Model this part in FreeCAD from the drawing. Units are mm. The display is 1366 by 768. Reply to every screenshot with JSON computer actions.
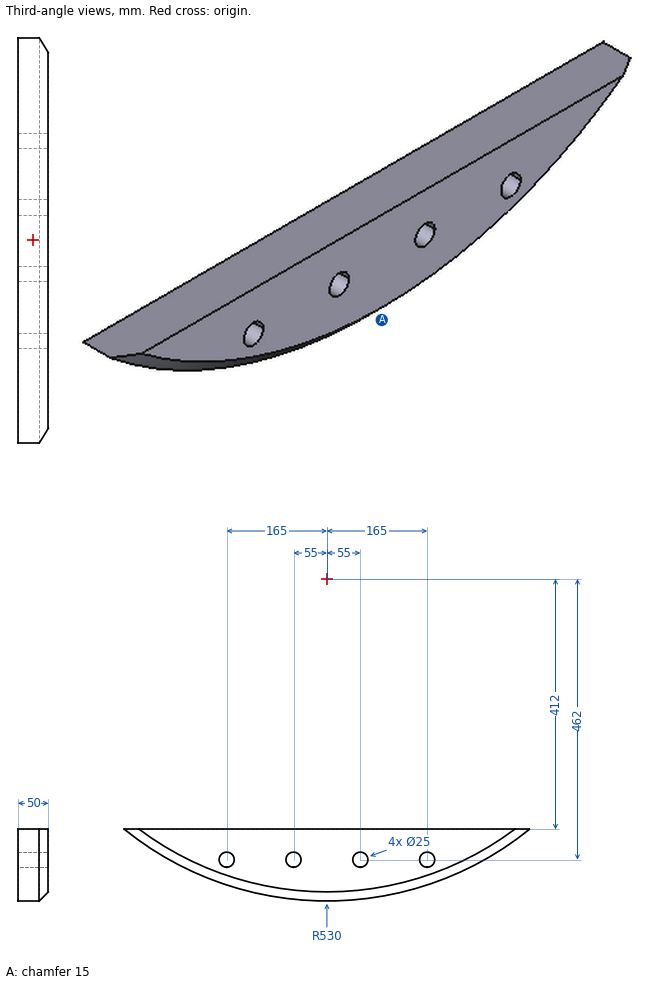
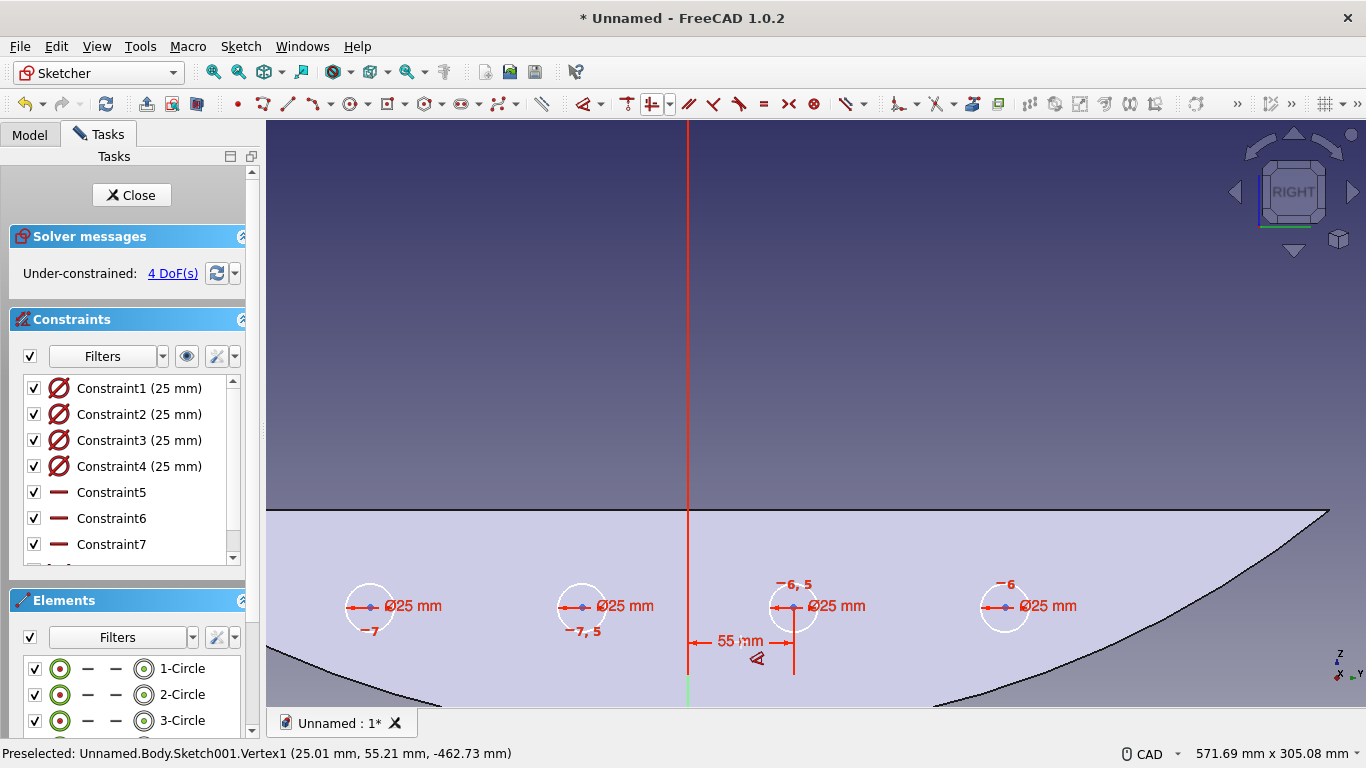
{"action": "left_click", "coordinate": [582, 608]}
{"action": "left_click", "coordinate": [635, 642]}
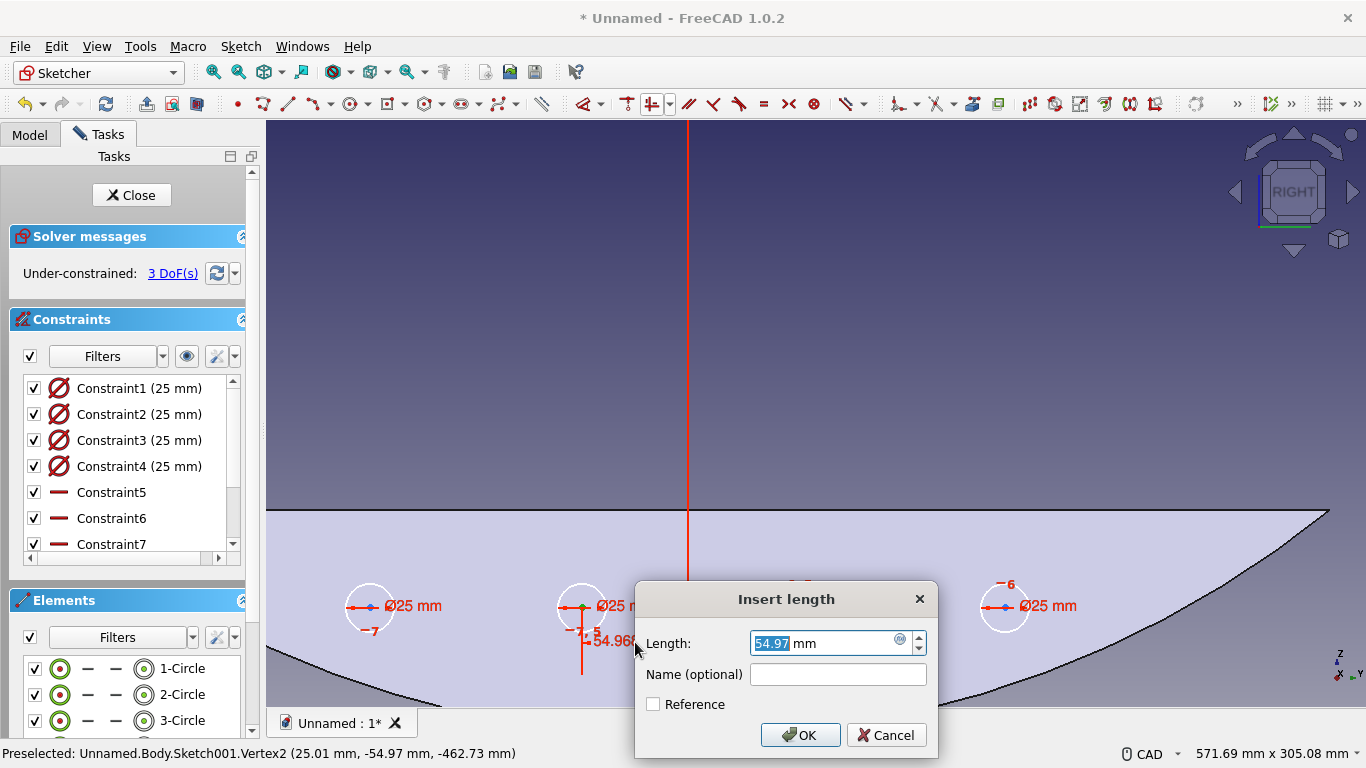
{"action": "type", "text": "55"}
{"action": "key", "text": "Return"}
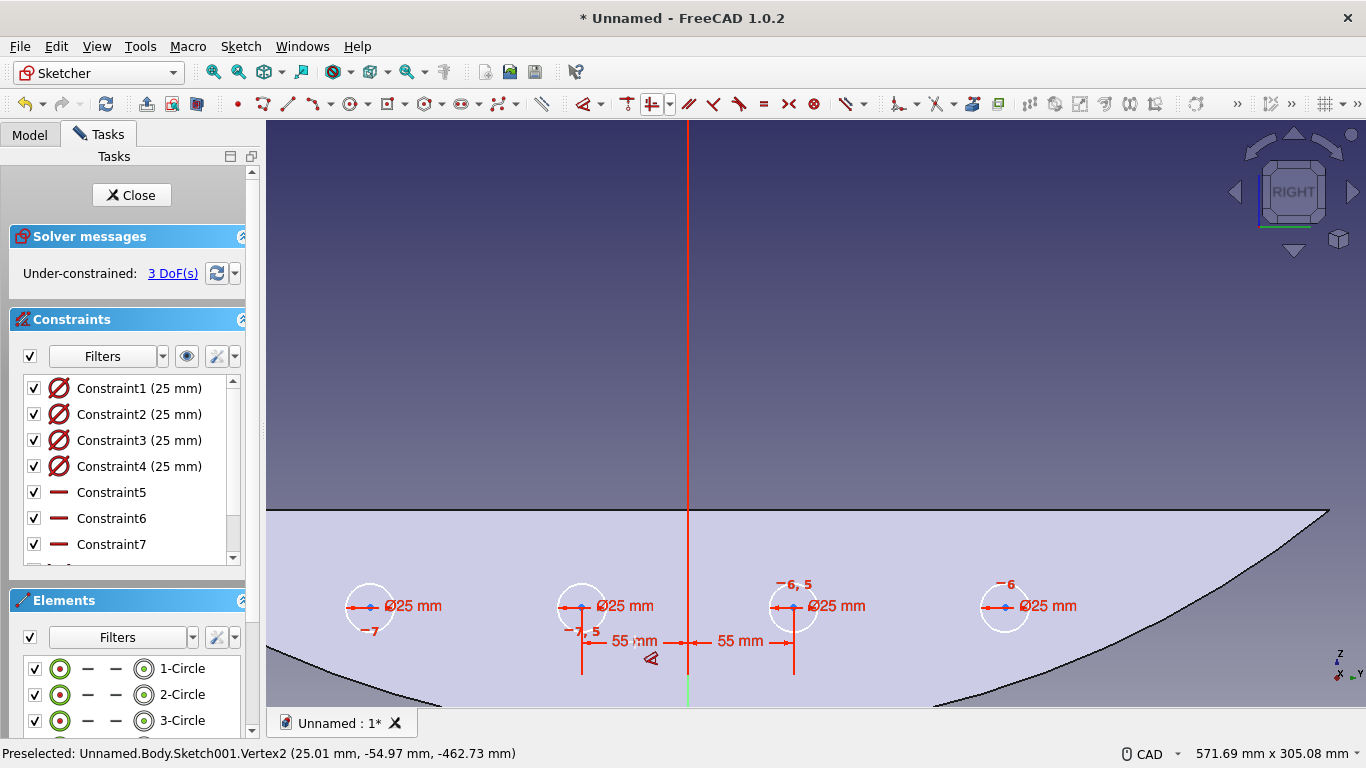
{"action": "left_click", "coordinate": [794, 608]}
{"action": "left_click", "coordinate": [828, 378]}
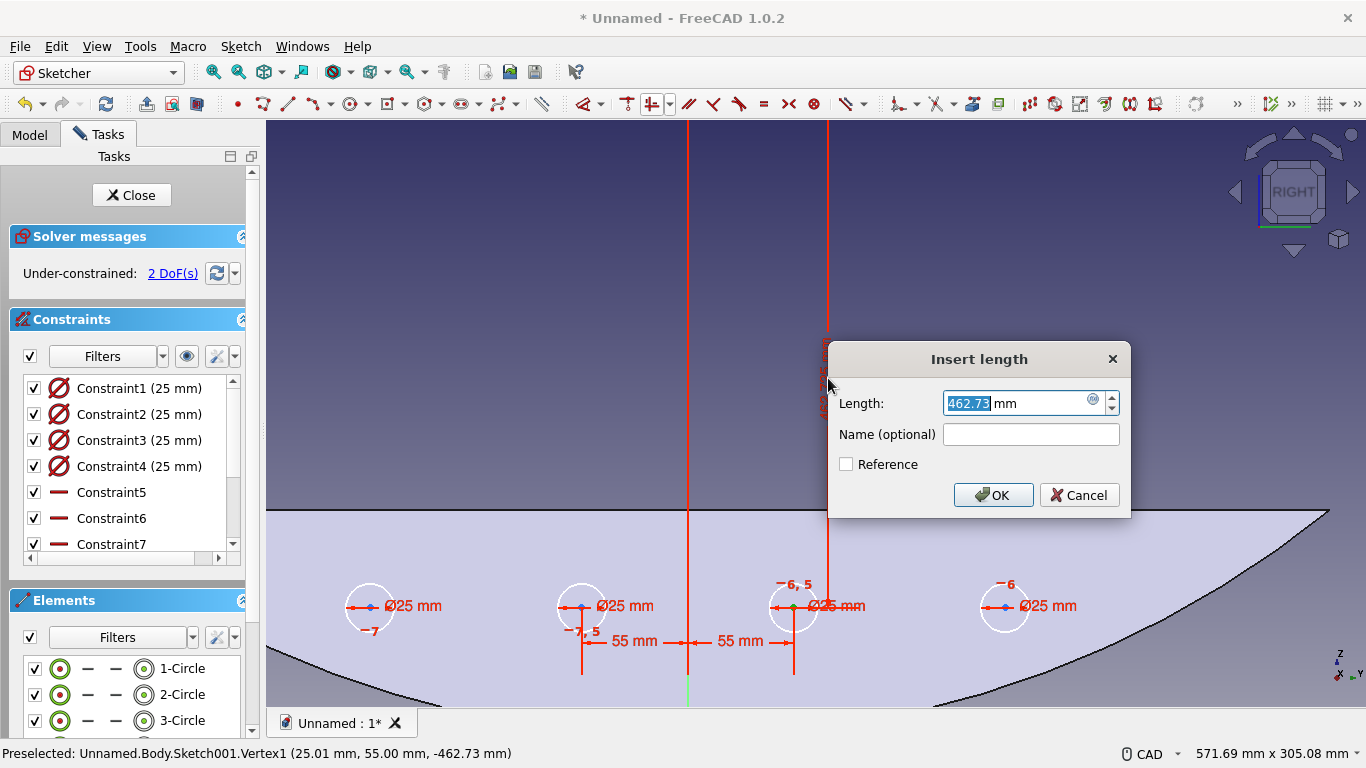
{"action": "type", "text": "462"}
{"action": "key", "text": "Return"}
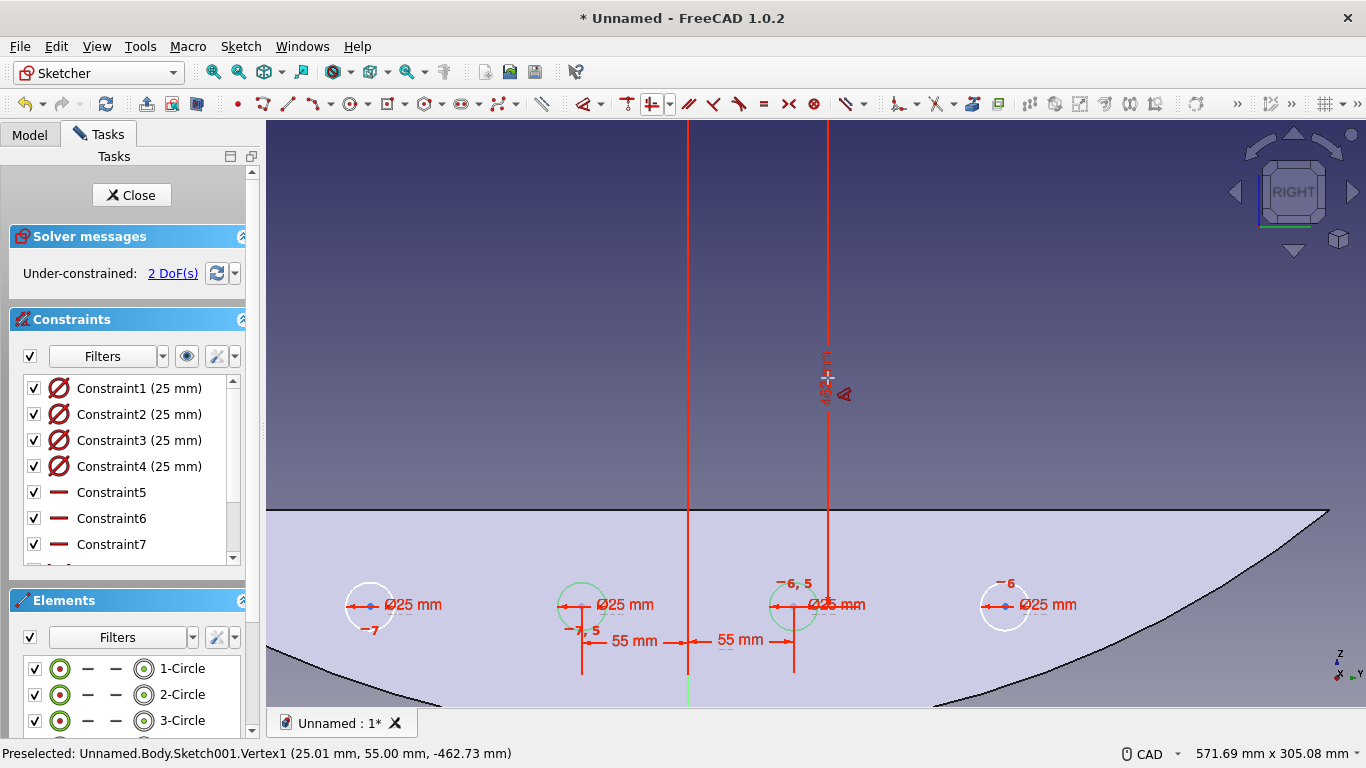
{"action": "left_click", "coordinate": [1005, 607]}
{"action": "left_click", "coordinate": [846, 641]}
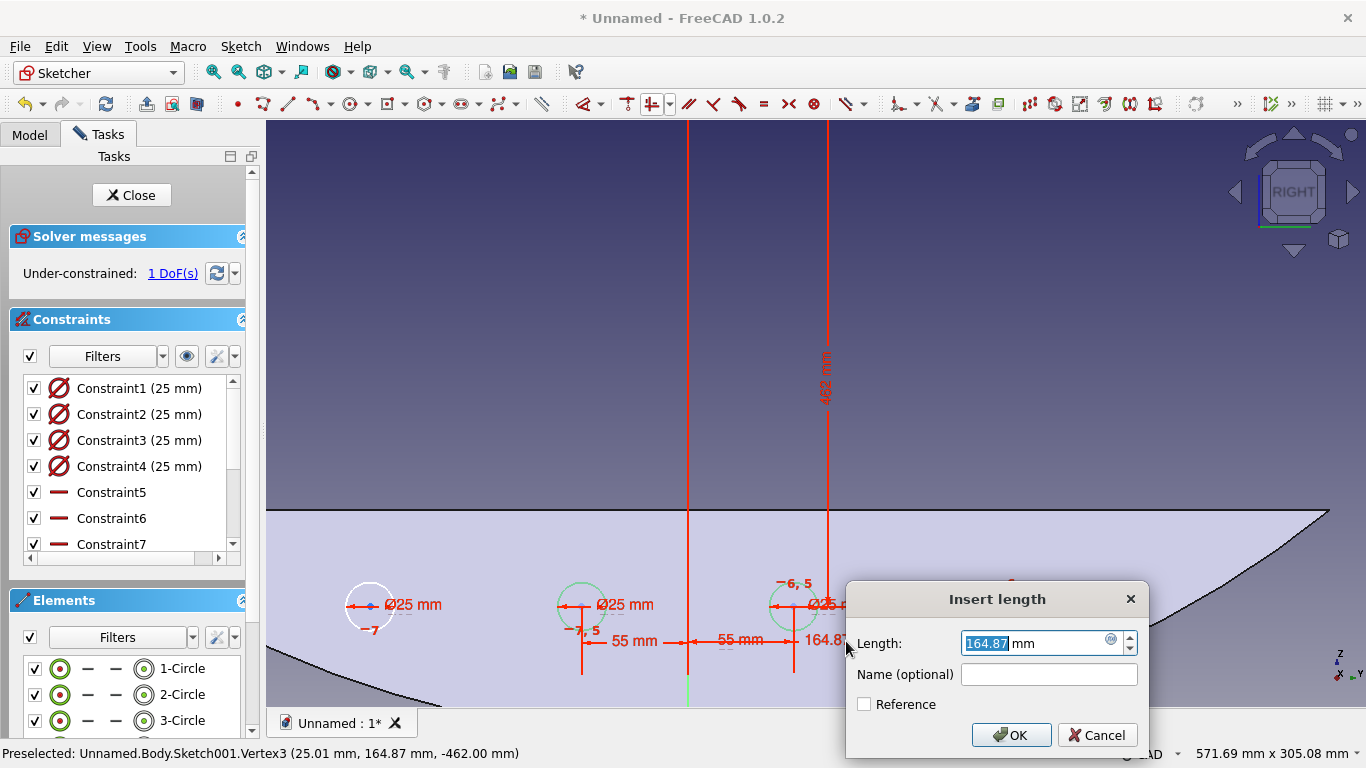
{"action": "type", "text": "165"}
{"action": "key", "text": "Return"}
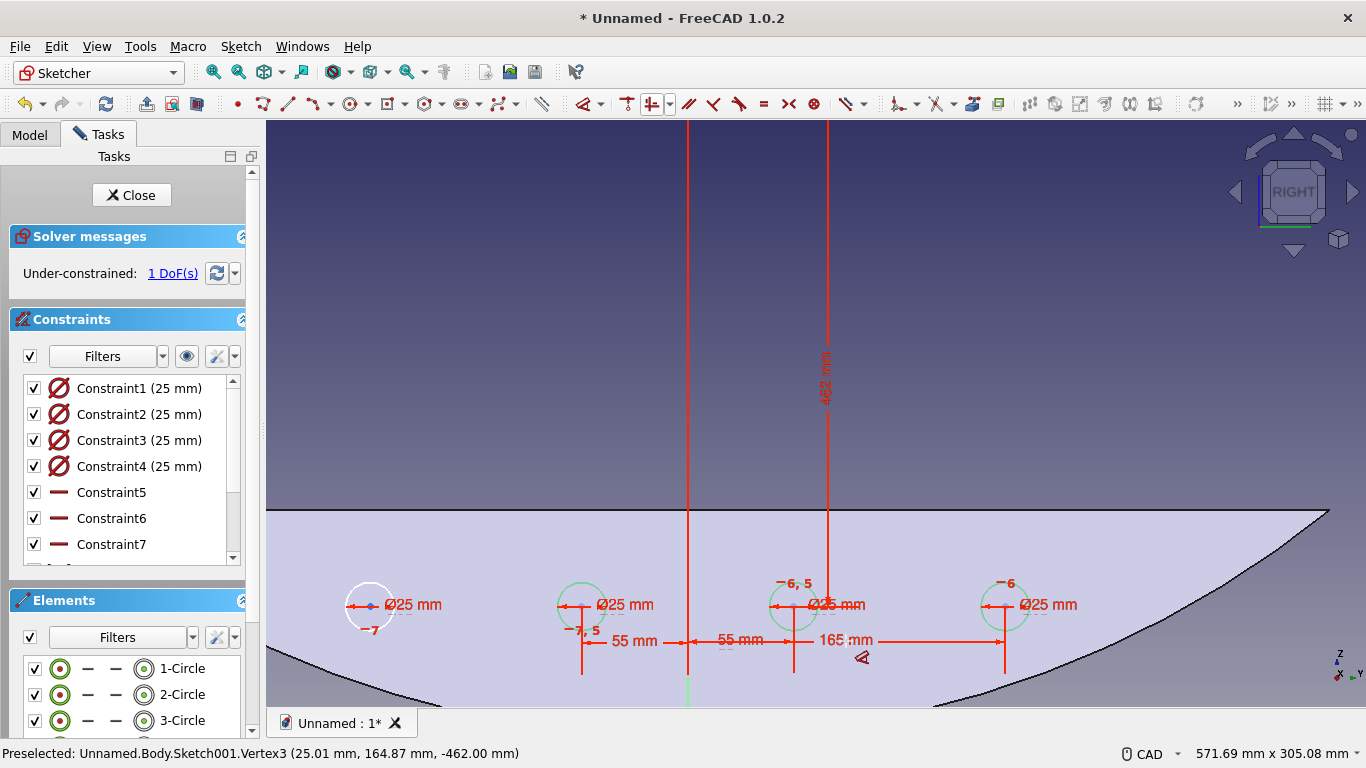
{"action": "left_click", "coordinate": [370, 607]}
{"action": "left_click", "coordinate": [529, 641]}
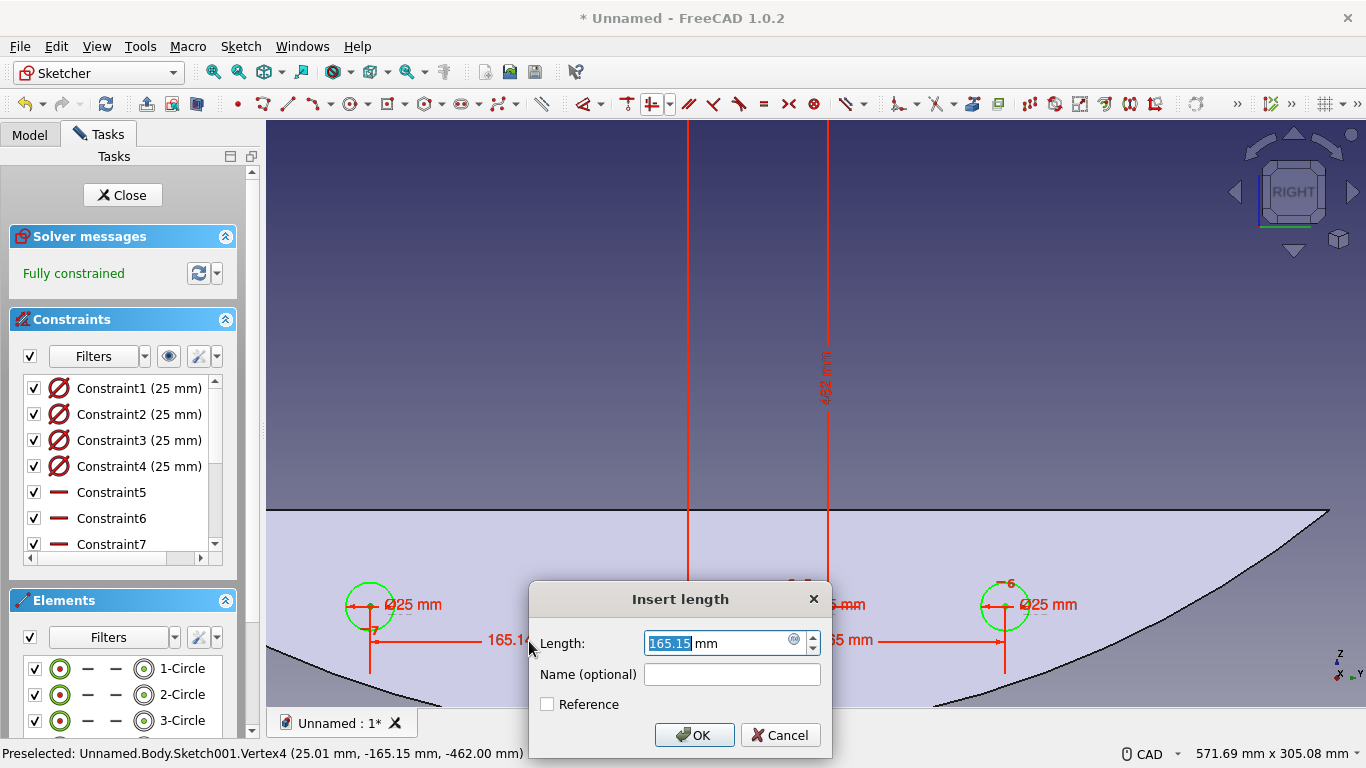
{"action": "type", "text": "165"}
{"action": "key", "text": "Return"}
{"action": "key", "text": "Escape"}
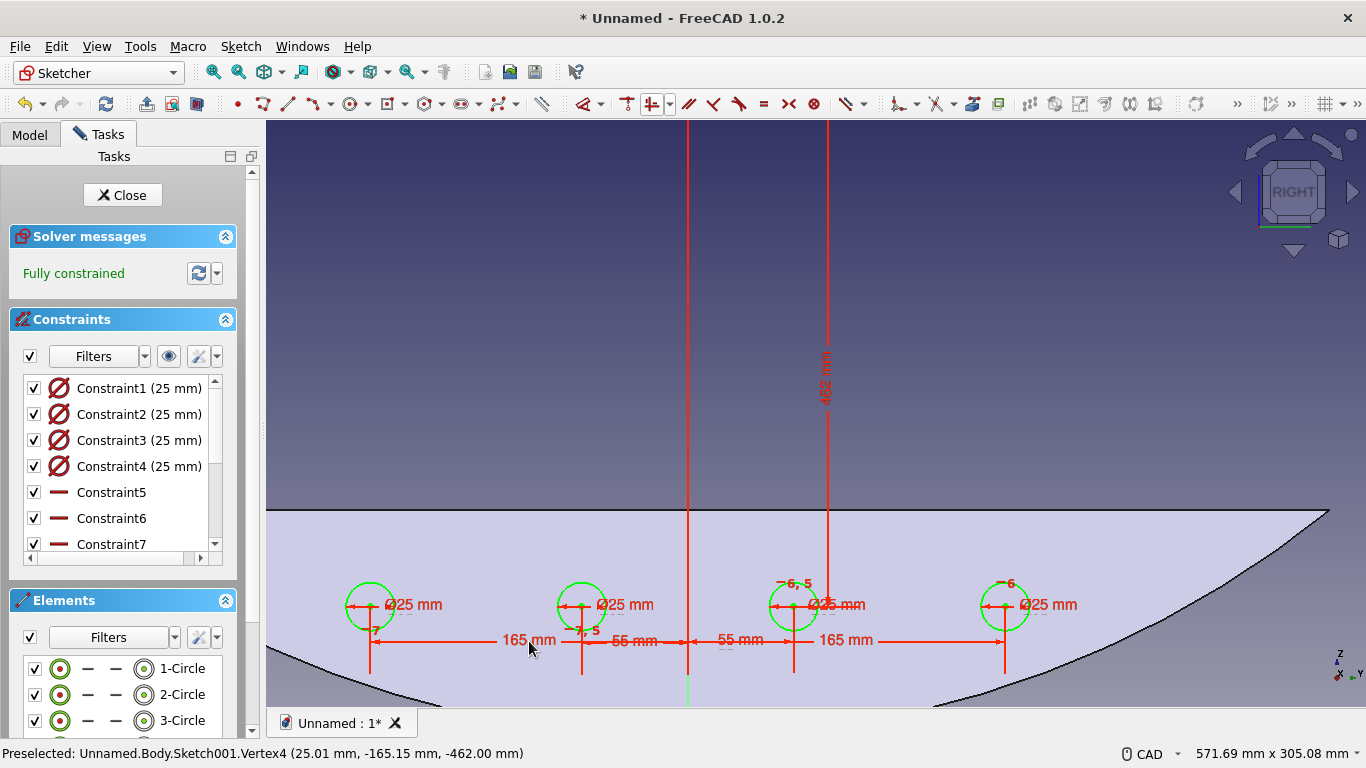
{"action": "left_click", "coordinate": [123, 195]}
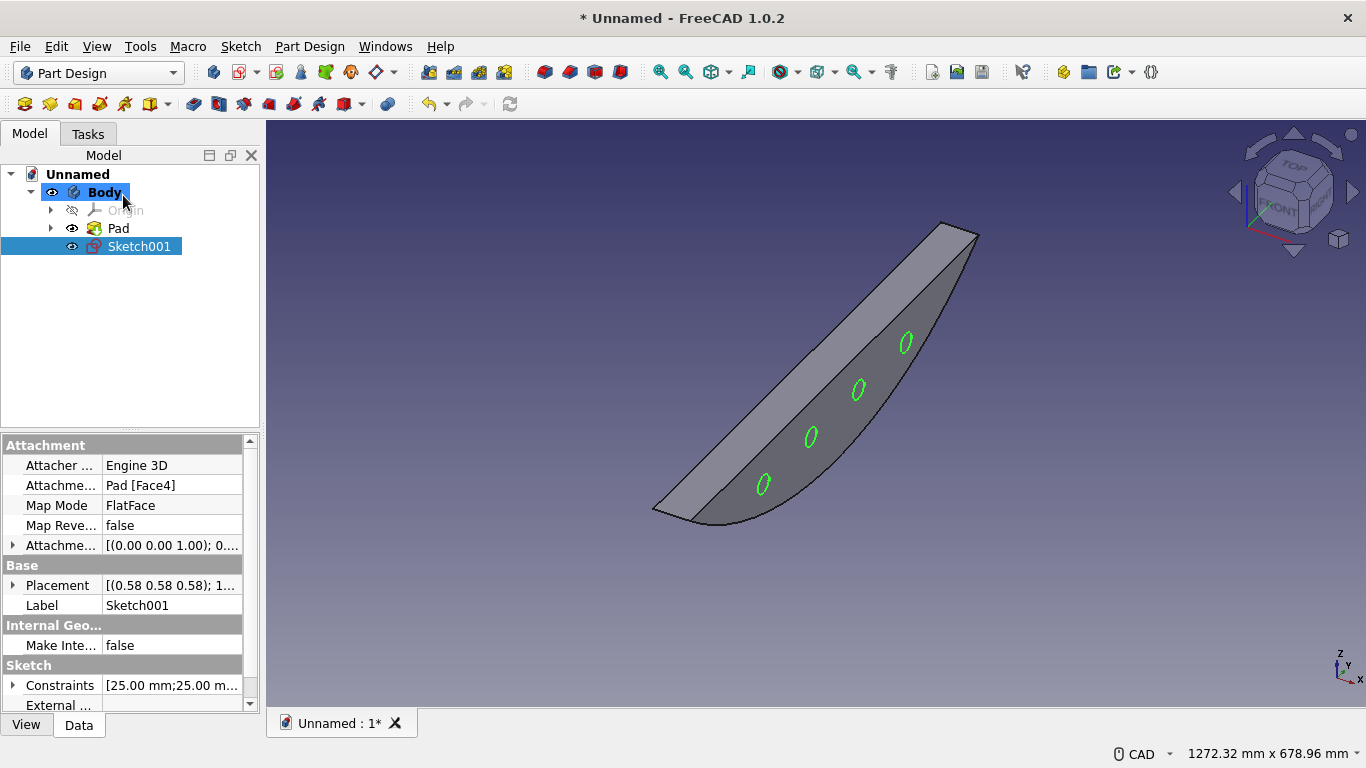
{"action": "left_click", "coordinate": [194, 104]}